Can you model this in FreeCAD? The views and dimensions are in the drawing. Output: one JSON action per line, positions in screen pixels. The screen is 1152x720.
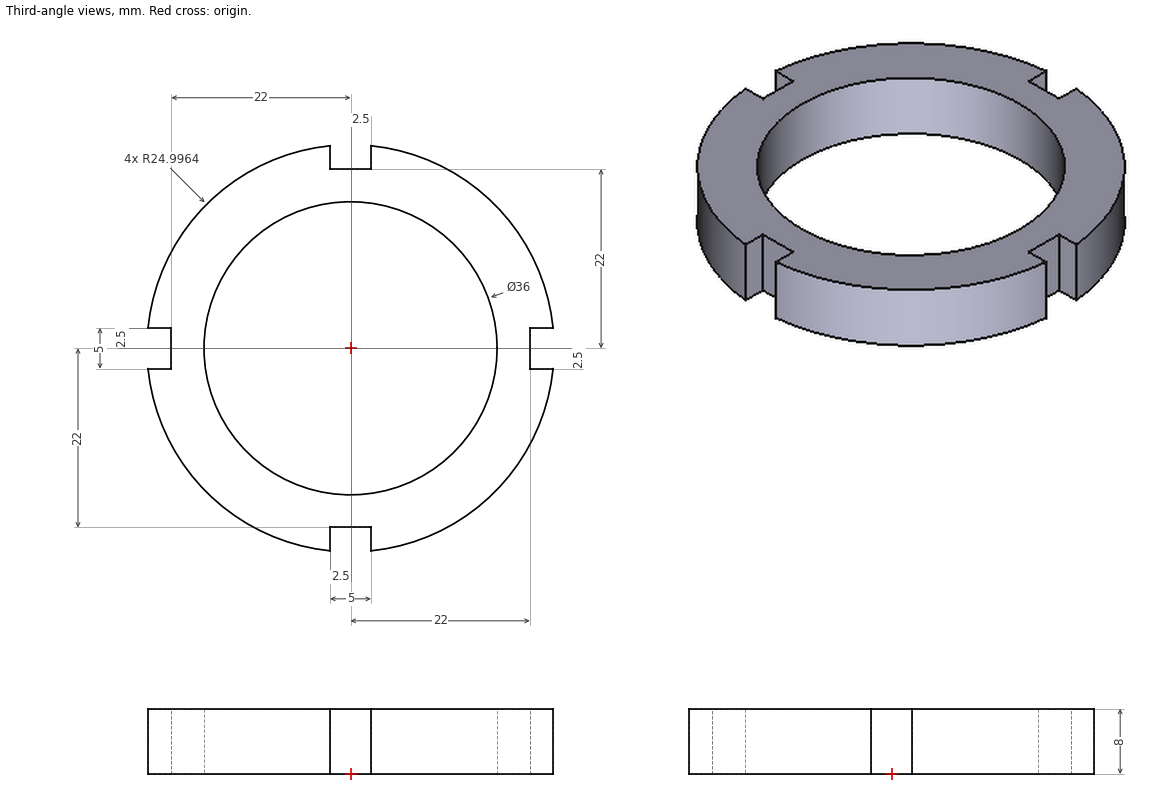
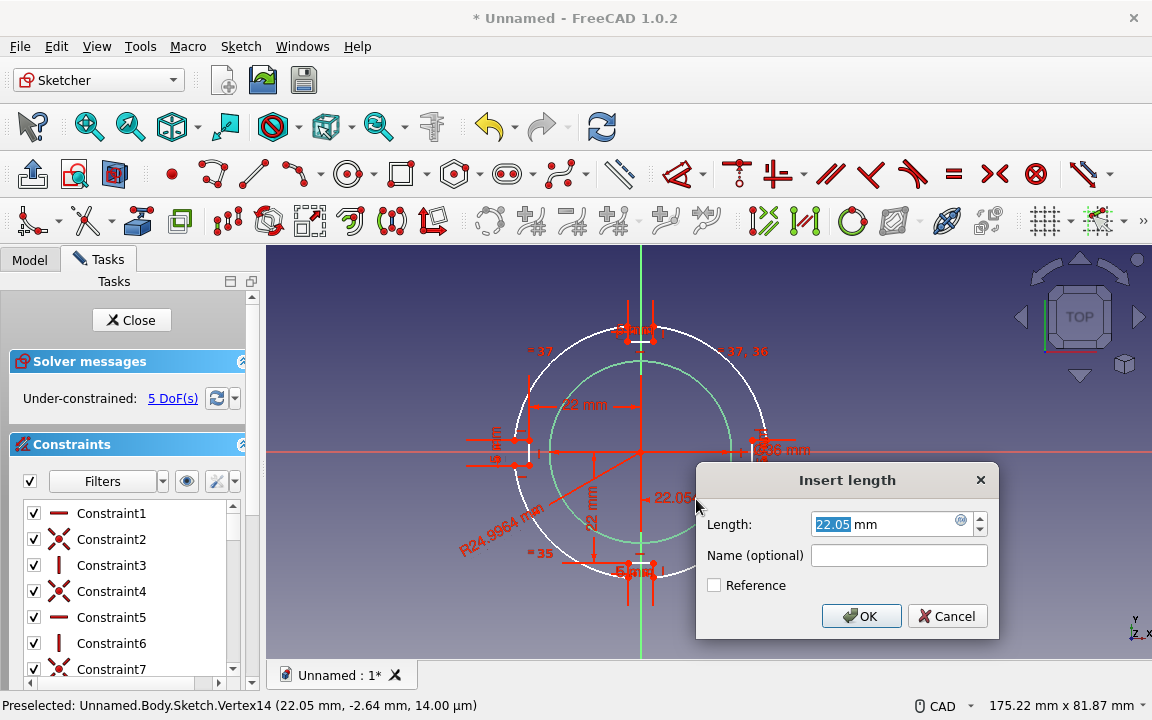
{"action": "type", "text": "22"}
{"action": "key", "text": "Return"}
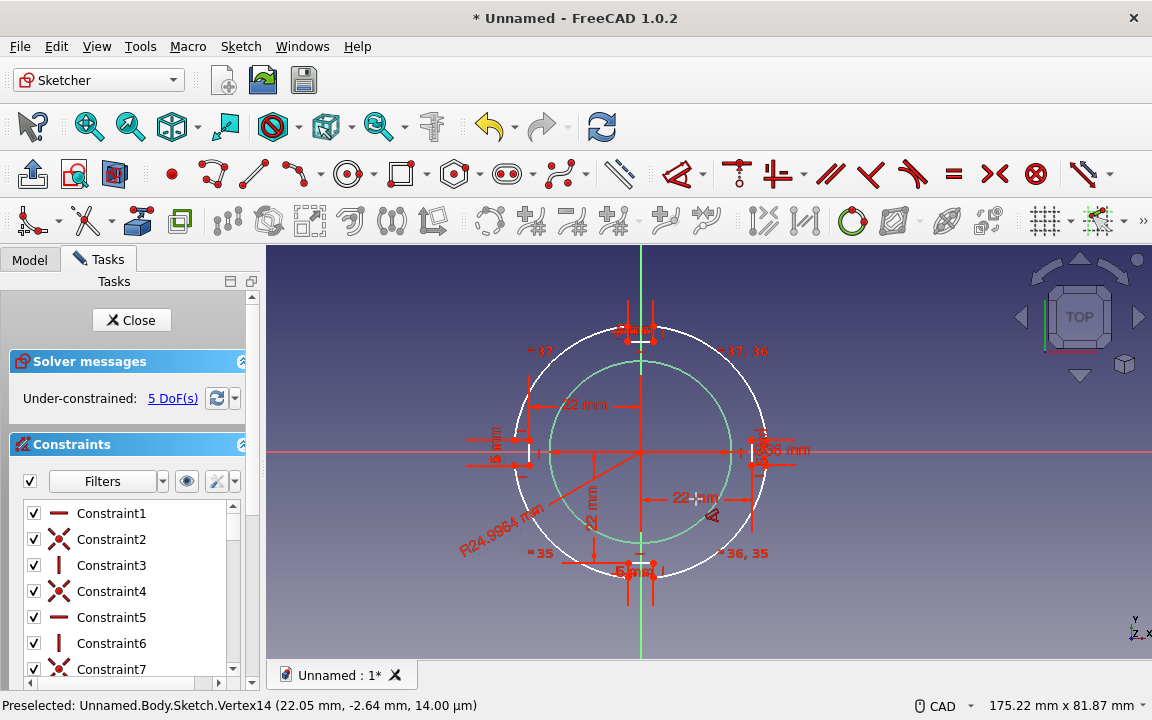
{"action": "left_click", "coordinate": [653, 342]}
{"action": "left_click", "coordinate": [687, 397]}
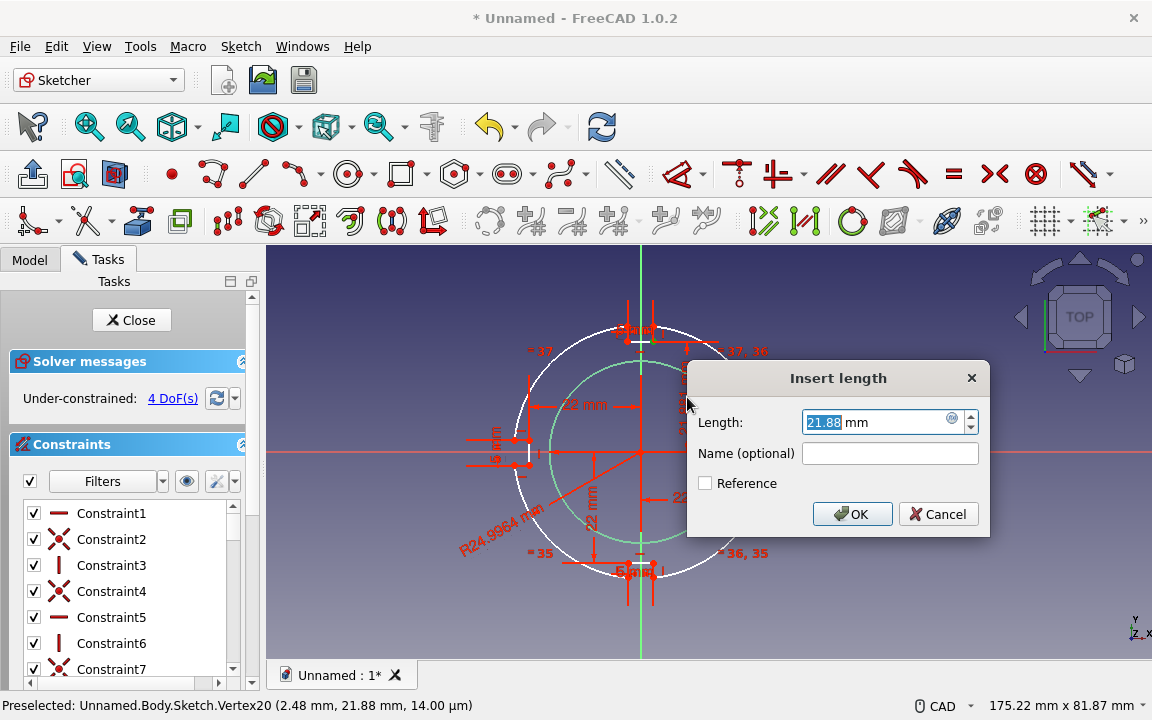
{"action": "type", "text": "22"}
{"action": "key", "text": "Return"}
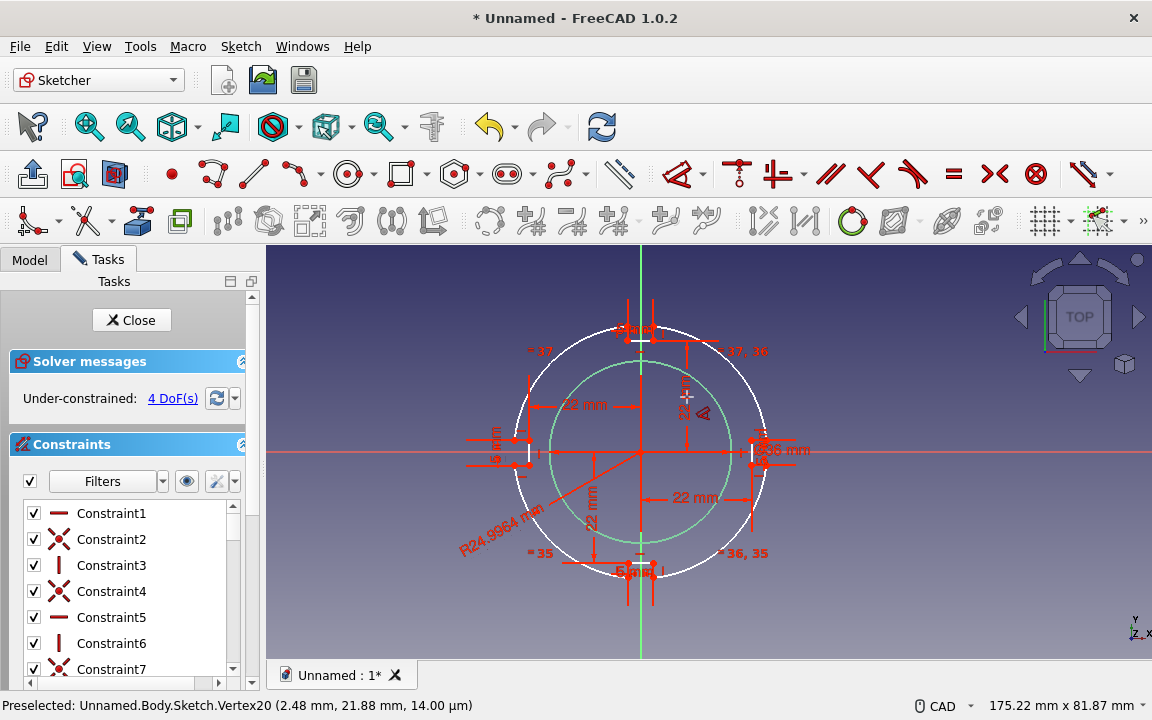
{"action": "scroll", "coordinate": [515, 440], "scroll_direction": "up", "scroll_amount": 6}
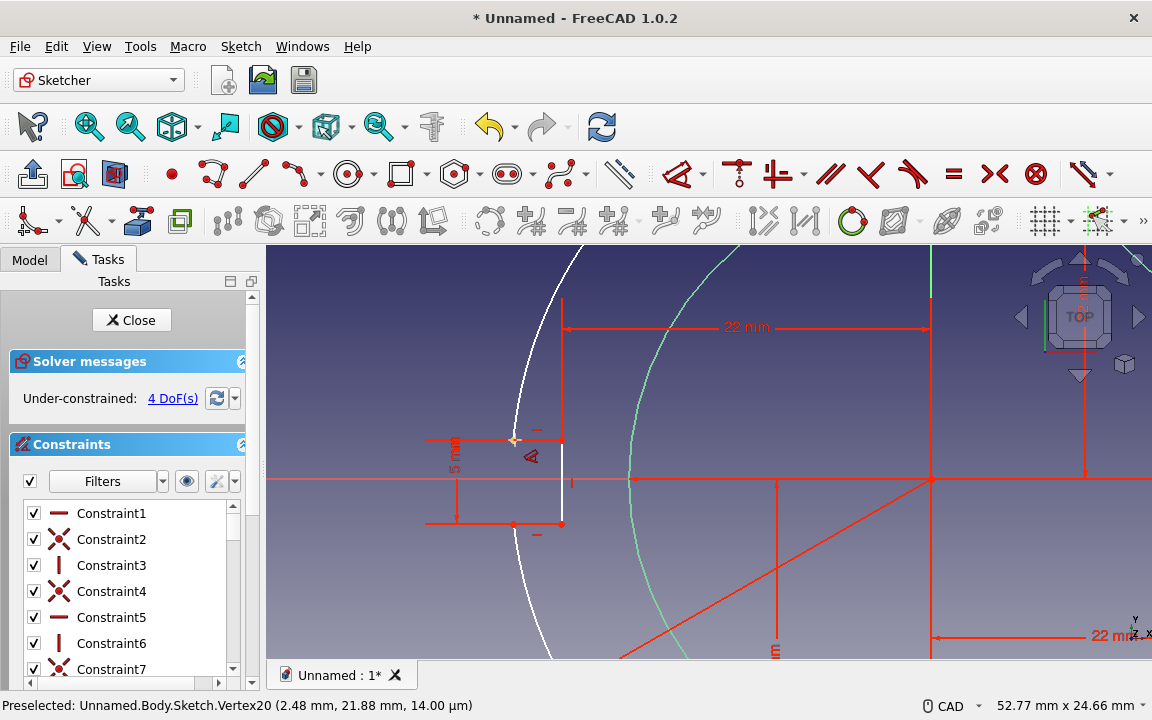
{"action": "left_click", "coordinate": [513, 440]}
{"action": "left_click", "coordinate": [965, 460]}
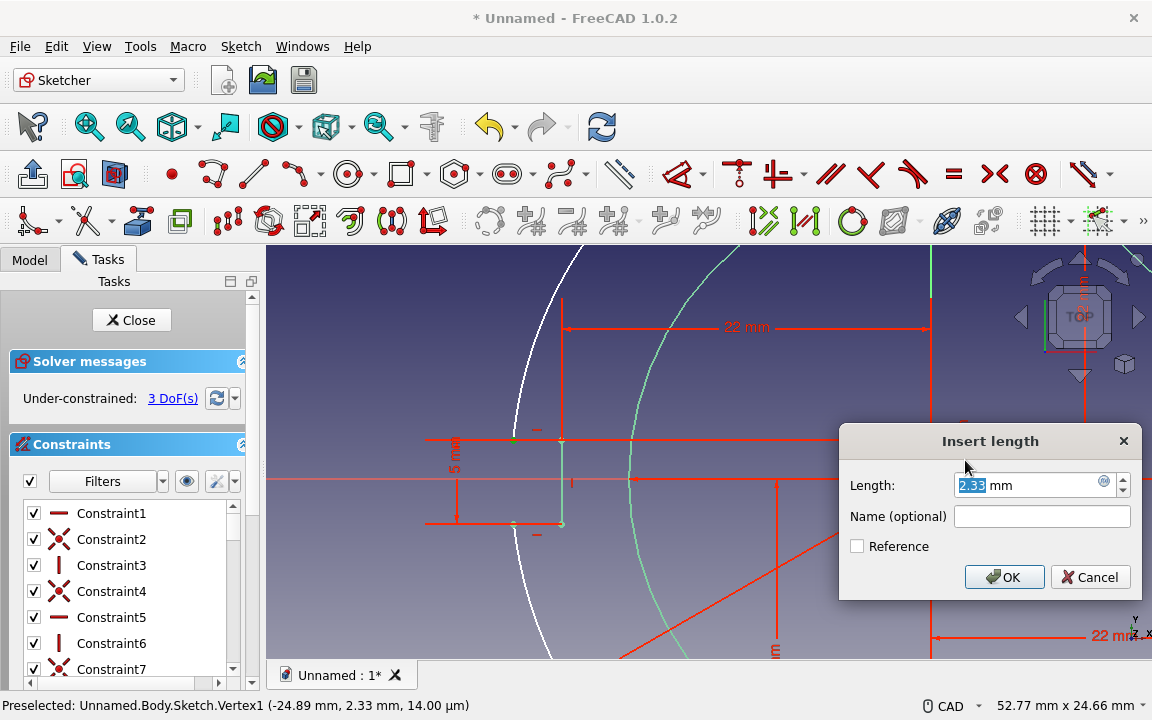
{"action": "type", "text": "2.5"}
{"action": "key", "text": "Return"}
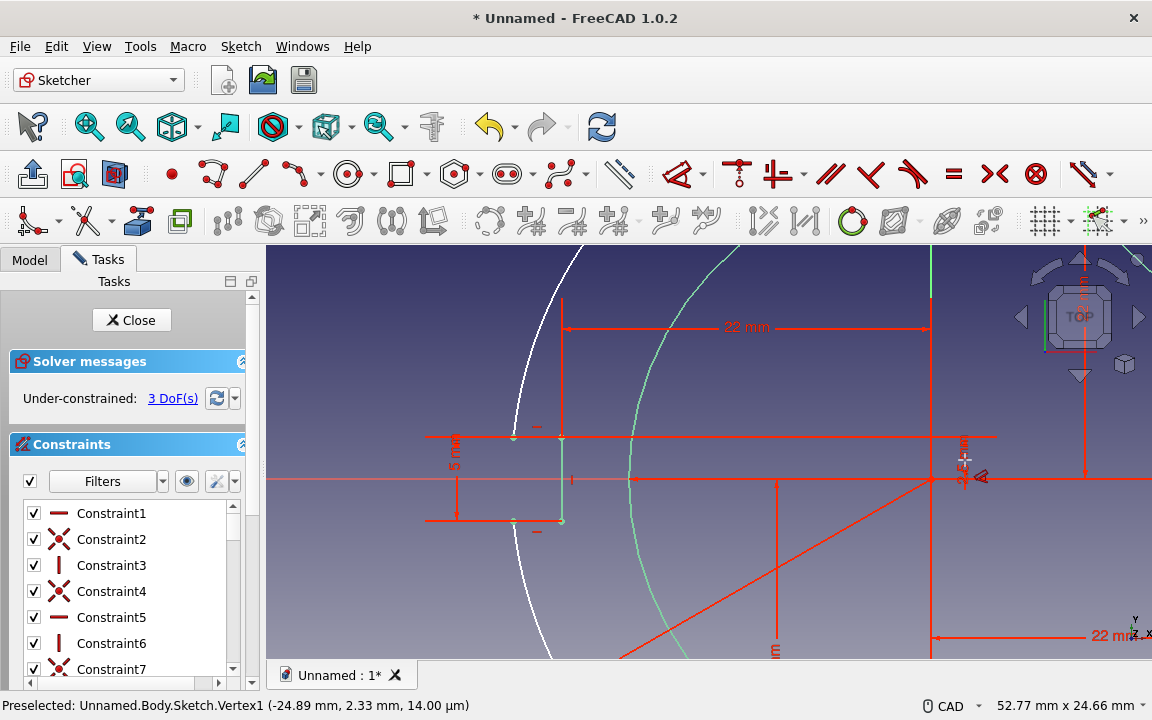
{"action": "scroll", "coordinate": [515, 440], "scroll_direction": "down", "scroll_amount": 6}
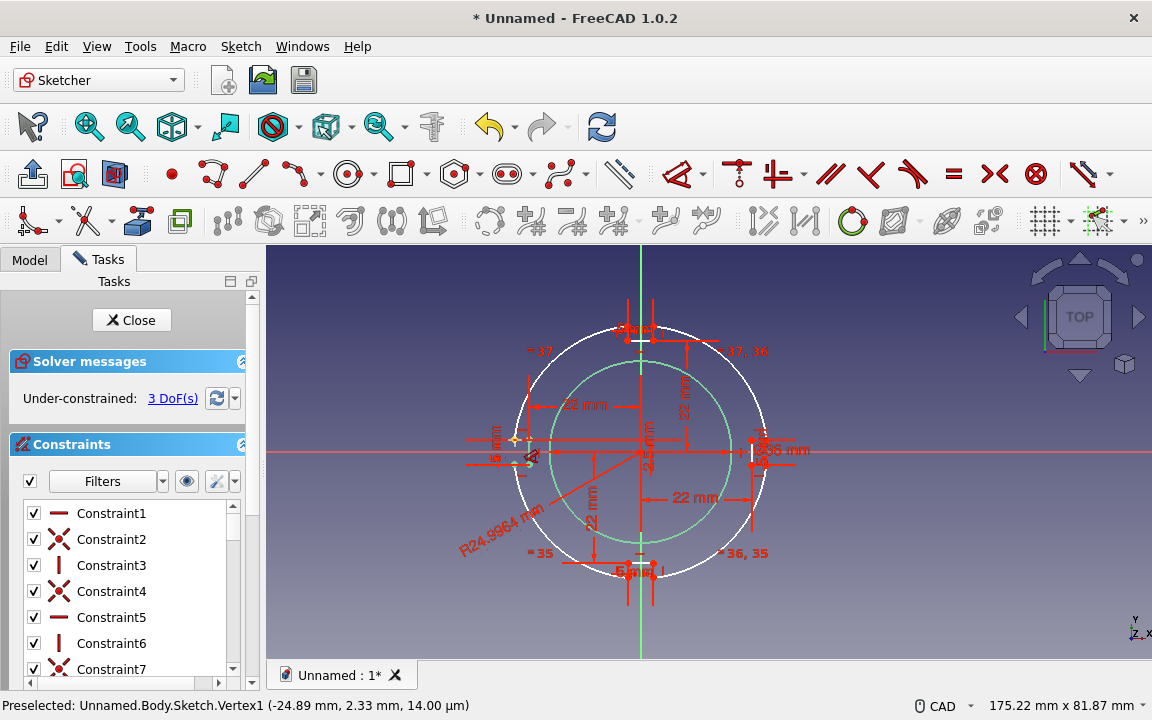
{"action": "scroll", "coordinate": [628, 578], "scroll_direction": "up", "scroll_amount": 6}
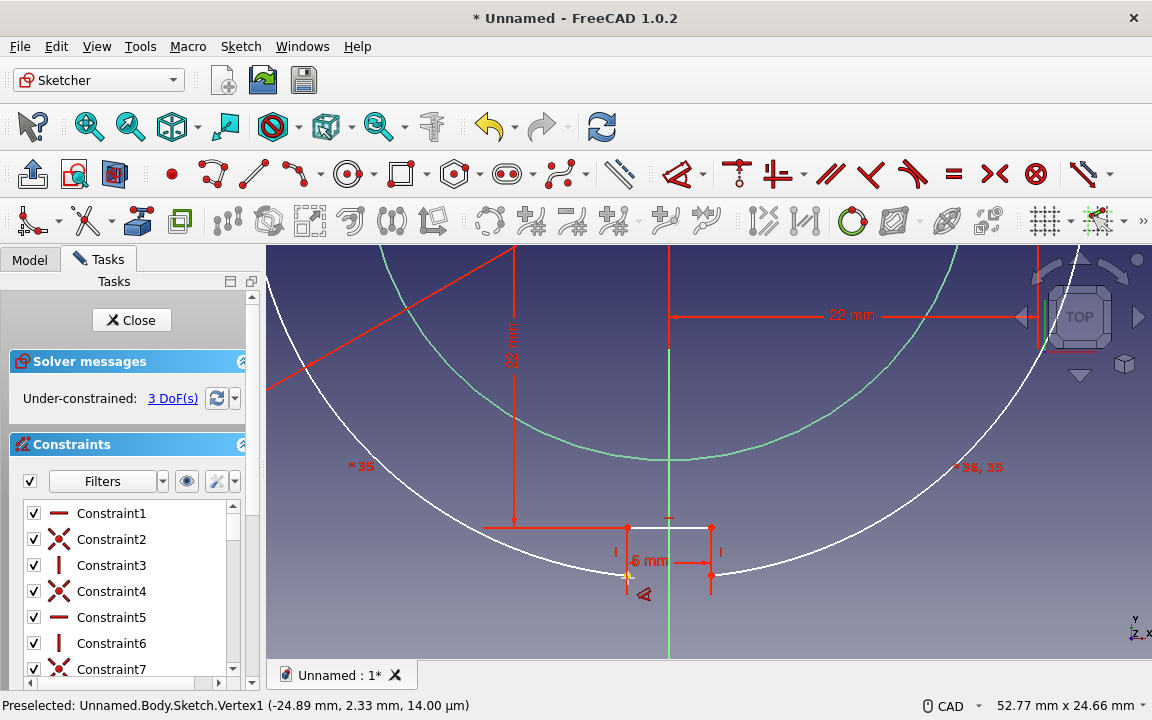
{"action": "left_click", "coordinate": [627, 576]}
{"action": "left_click", "coordinate": [648, 610]}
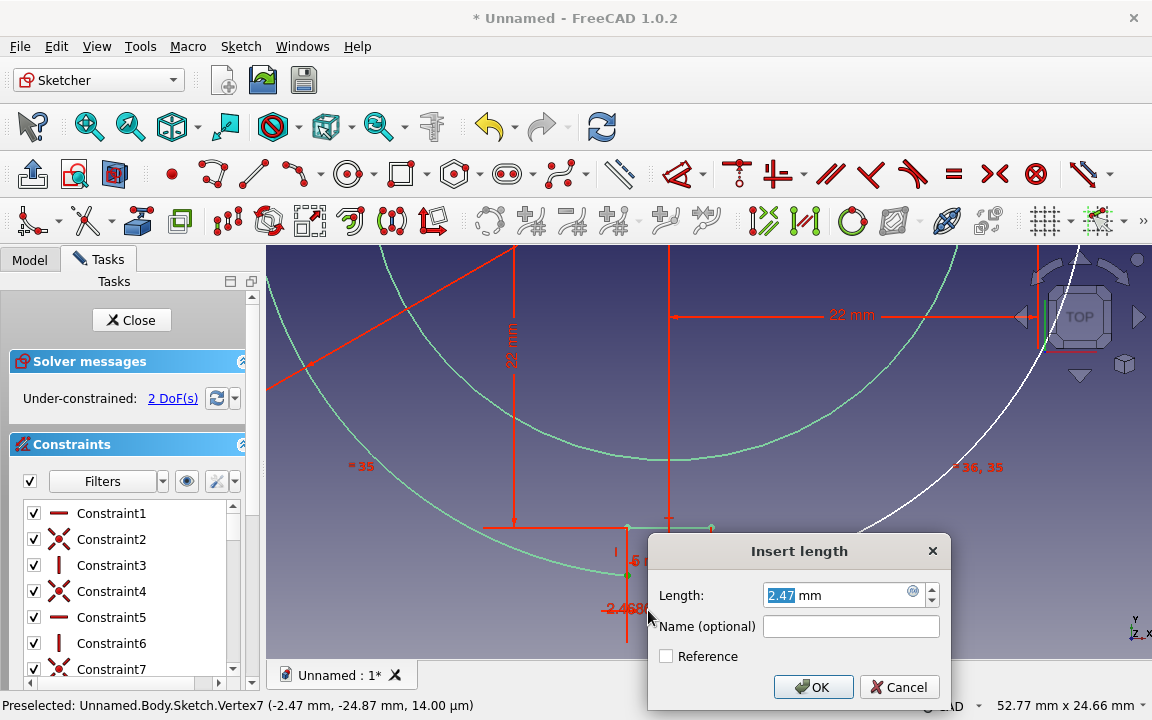
{"action": "type", "text": "2.5"}
{"action": "key", "text": "Return"}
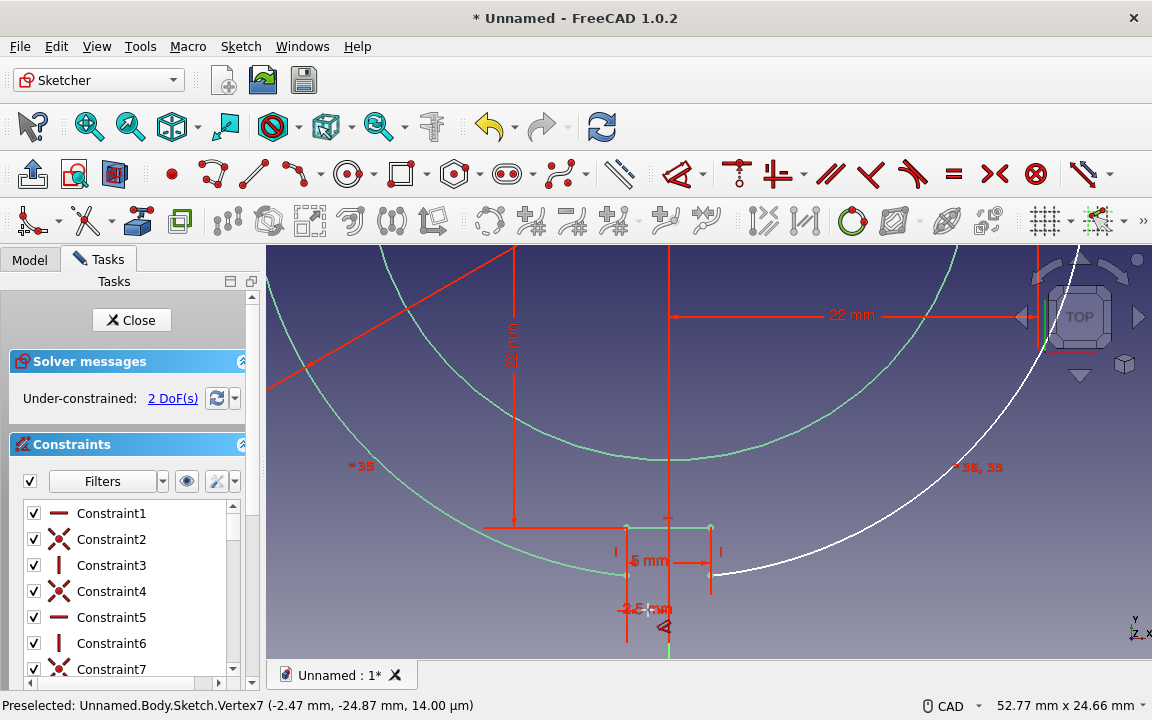
{"action": "scroll", "coordinate": [628, 579], "scroll_direction": "down", "scroll_amount": 6}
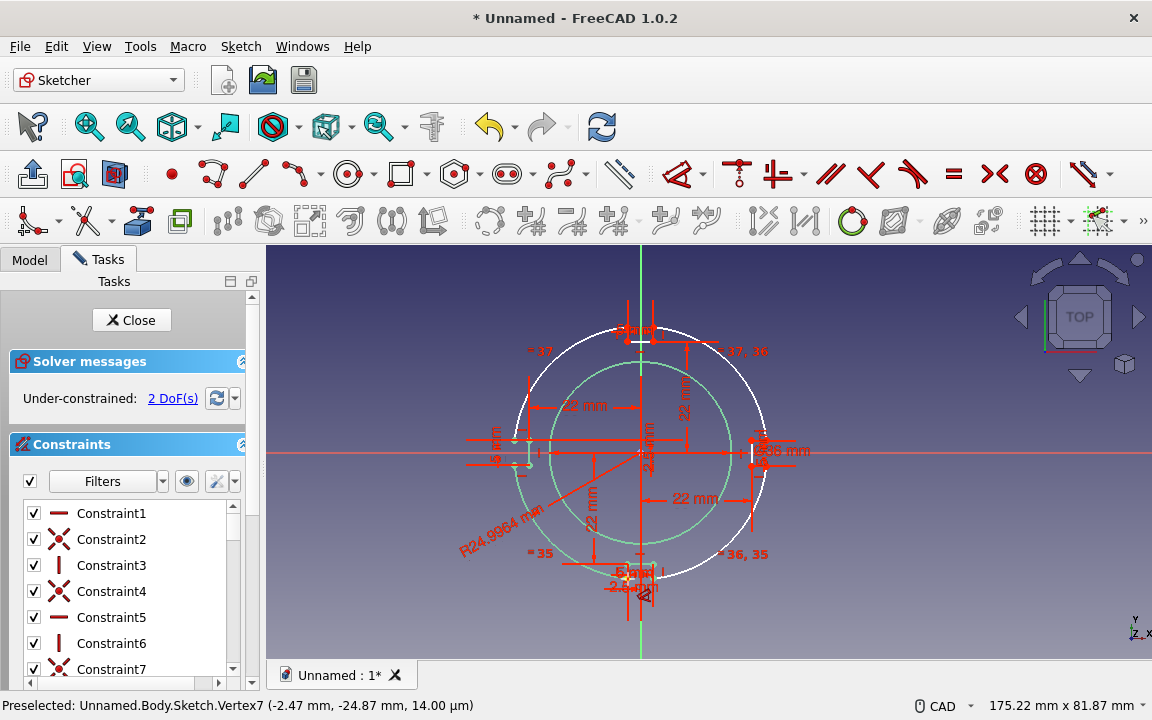
{"action": "scroll", "coordinate": [766, 466], "scroll_direction": "up", "scroll_amount": 6}